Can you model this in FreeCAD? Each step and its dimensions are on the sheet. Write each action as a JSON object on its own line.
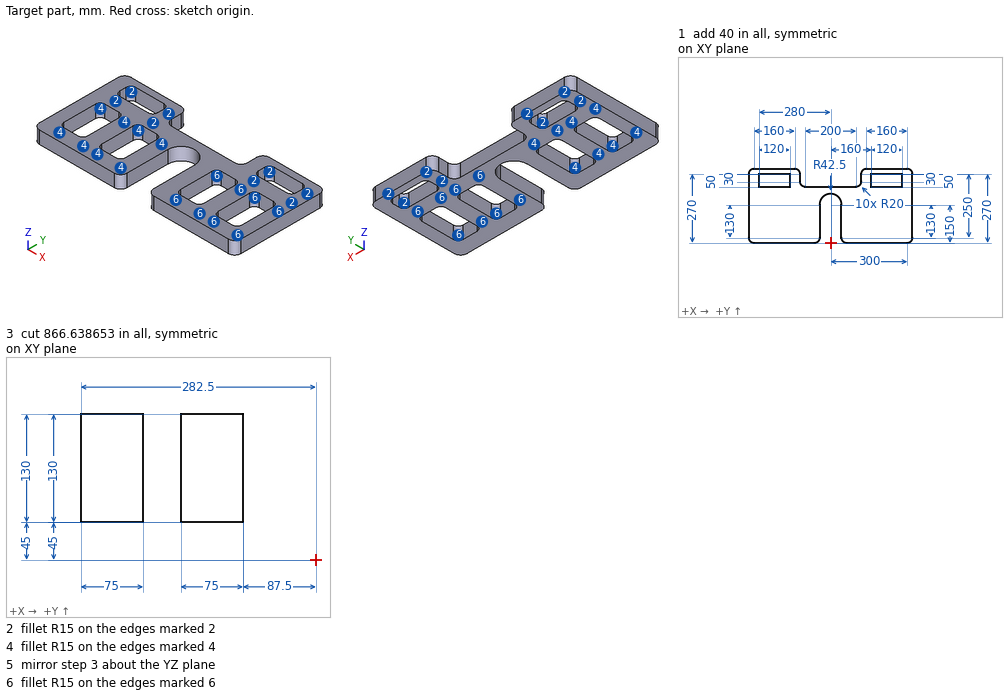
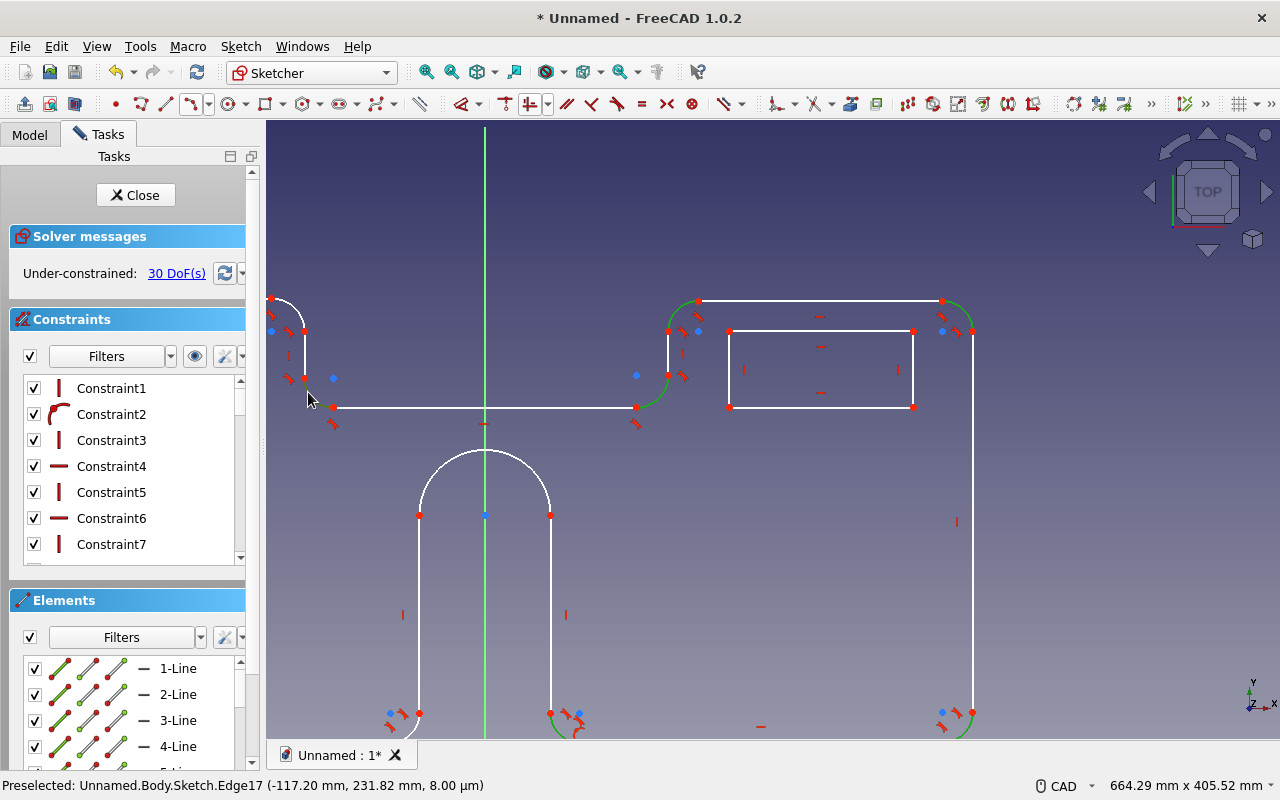
{"action": "left_click", "coordinate": [301, 316]}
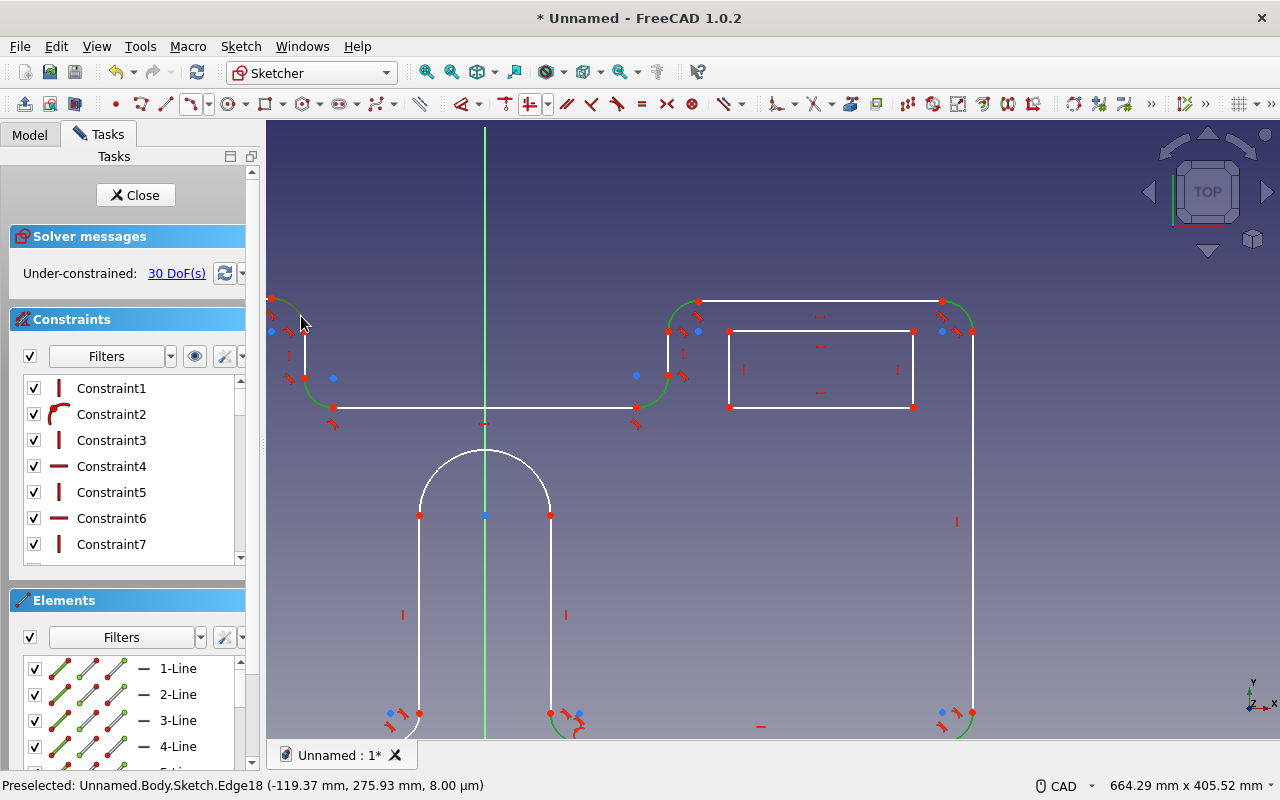
{"action": "scroll", "coordinate": [971, 318], "scroll_direction": "down", "scroll_amount": 3}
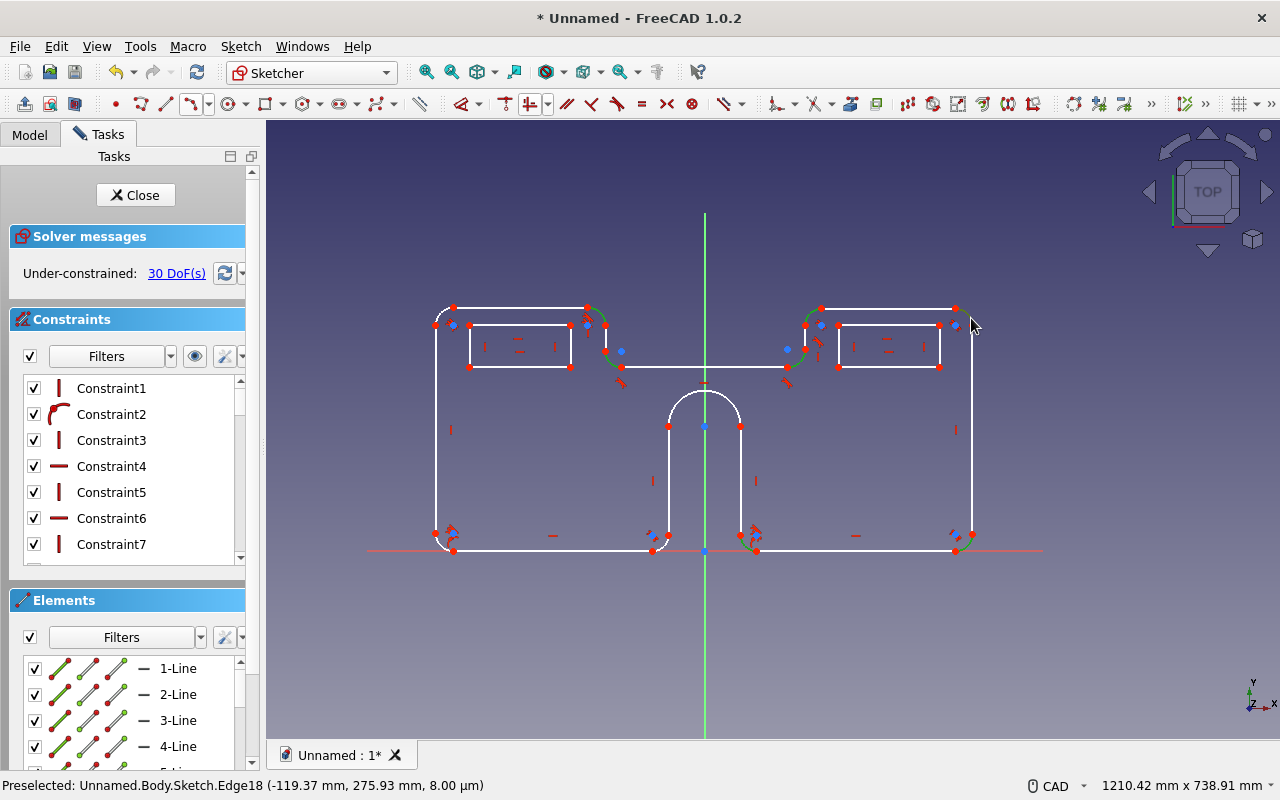
{"action": "scroll", "coordinate": [446, 309], "scroll_direction": "up", "scroll_amount": 3}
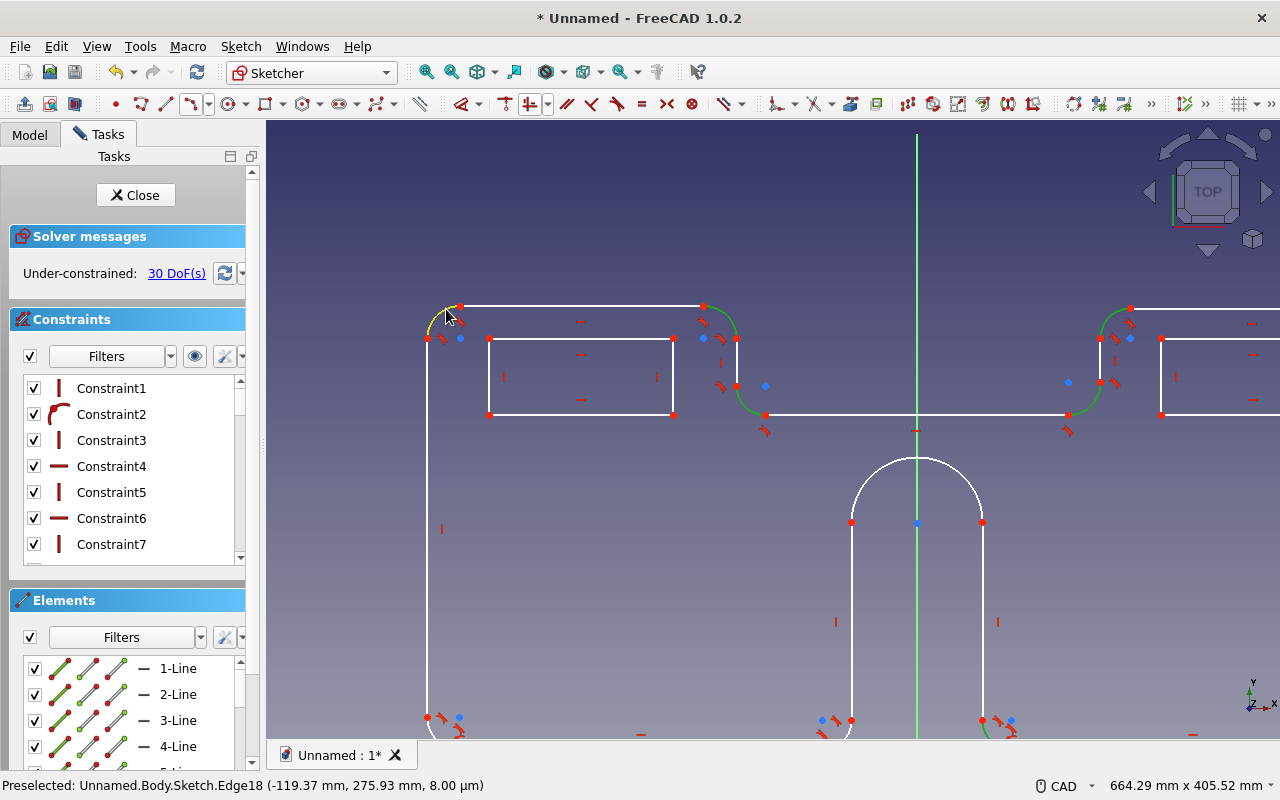
{"action": "left_click", "coordinate": [445, 310]}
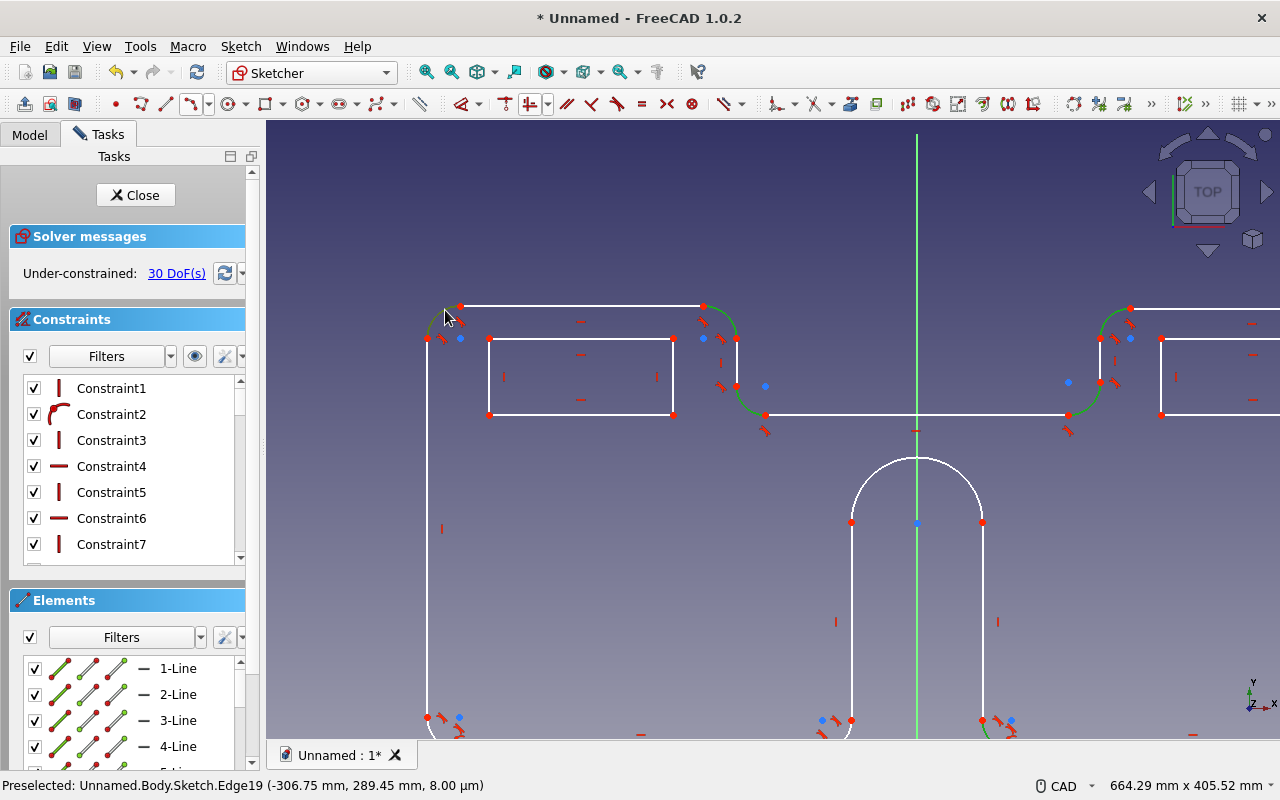
{"action": "scroll", "coordinate": [446, 309], "scroll_direction": "down", "scroll_amount": 3}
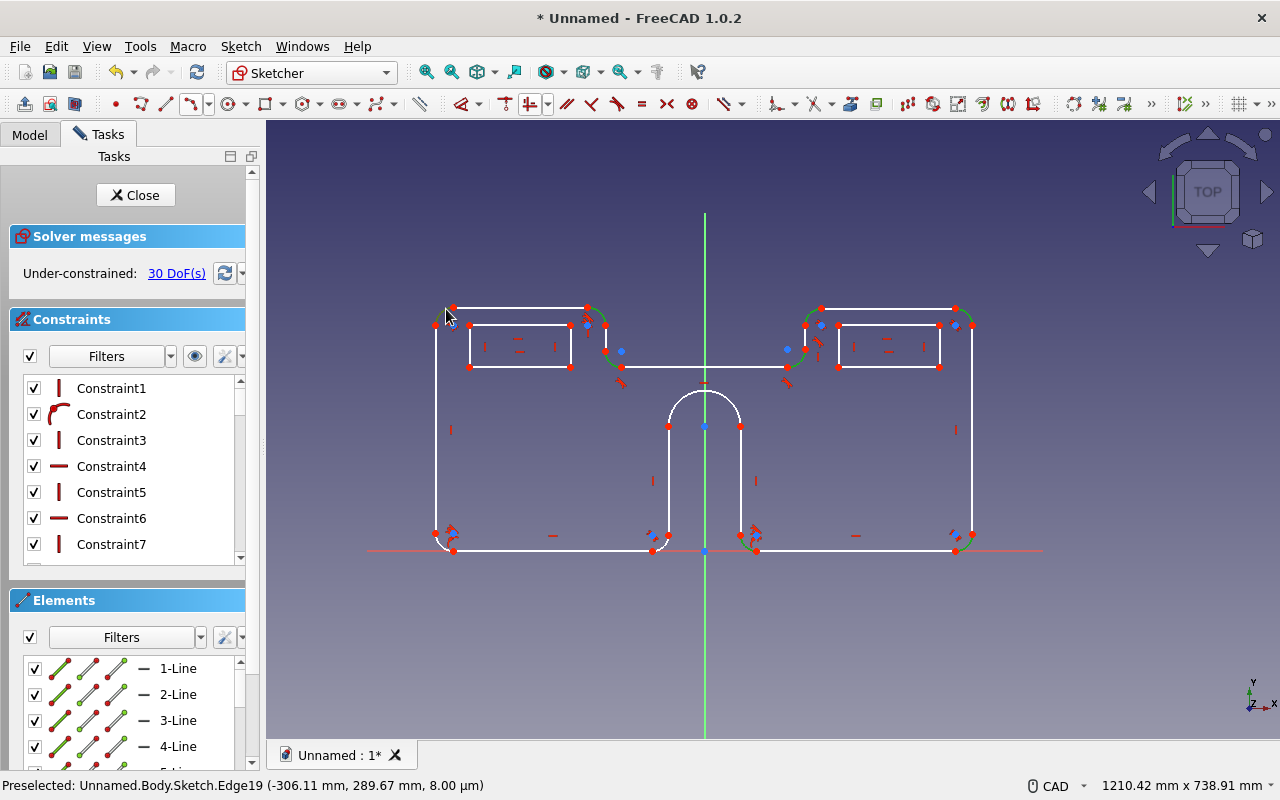
{"action": "scroll", "coordinate": [438, 541], "scroll_direction": "up", "scroll_amount": 3}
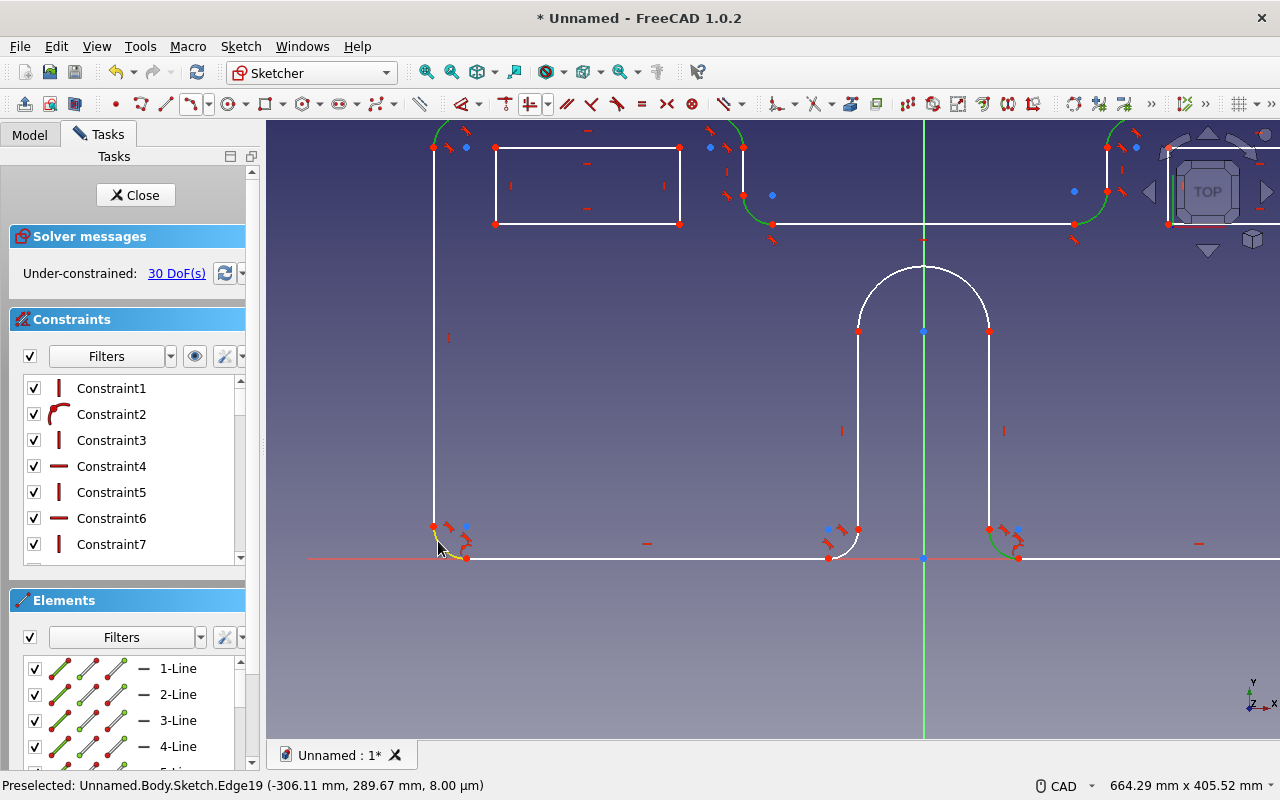
{"action": "left_click", "coordinate": [437, 541]}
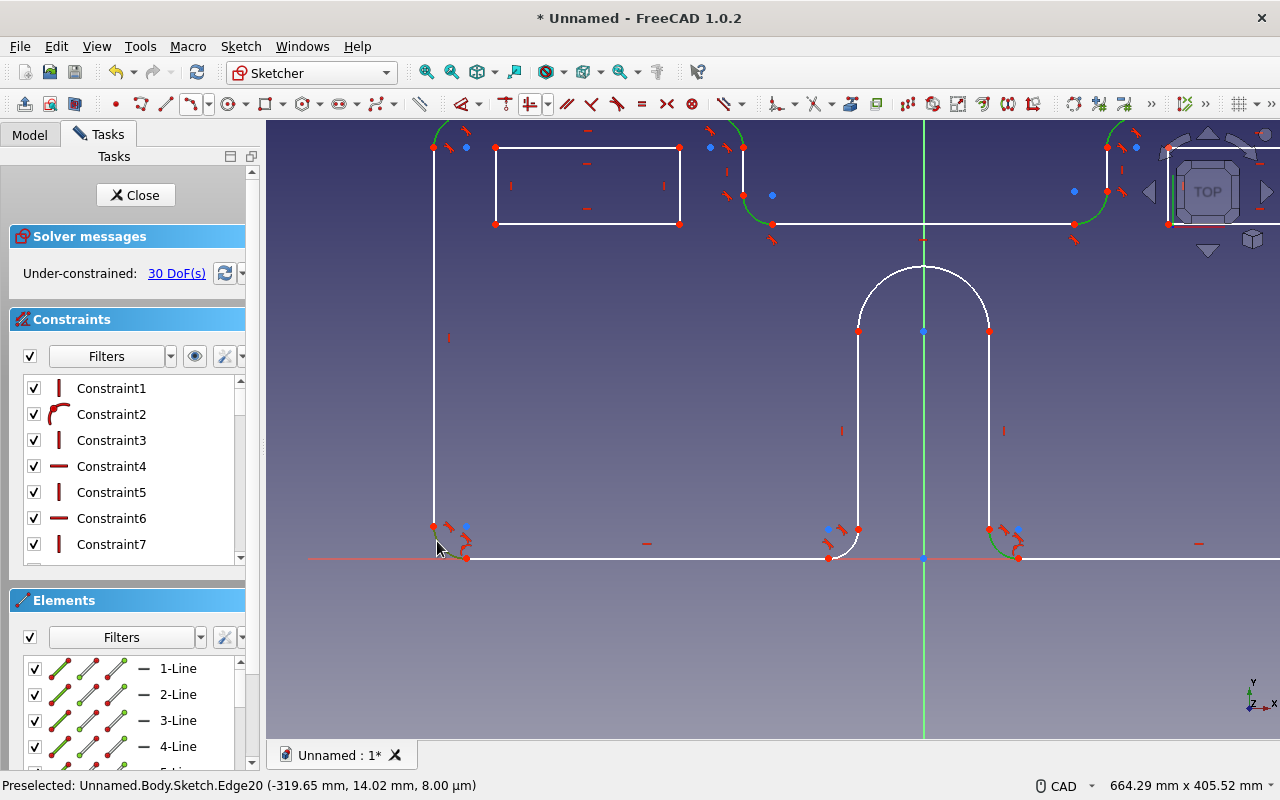
{"action": "left_click", "coordinate": [842, 556]}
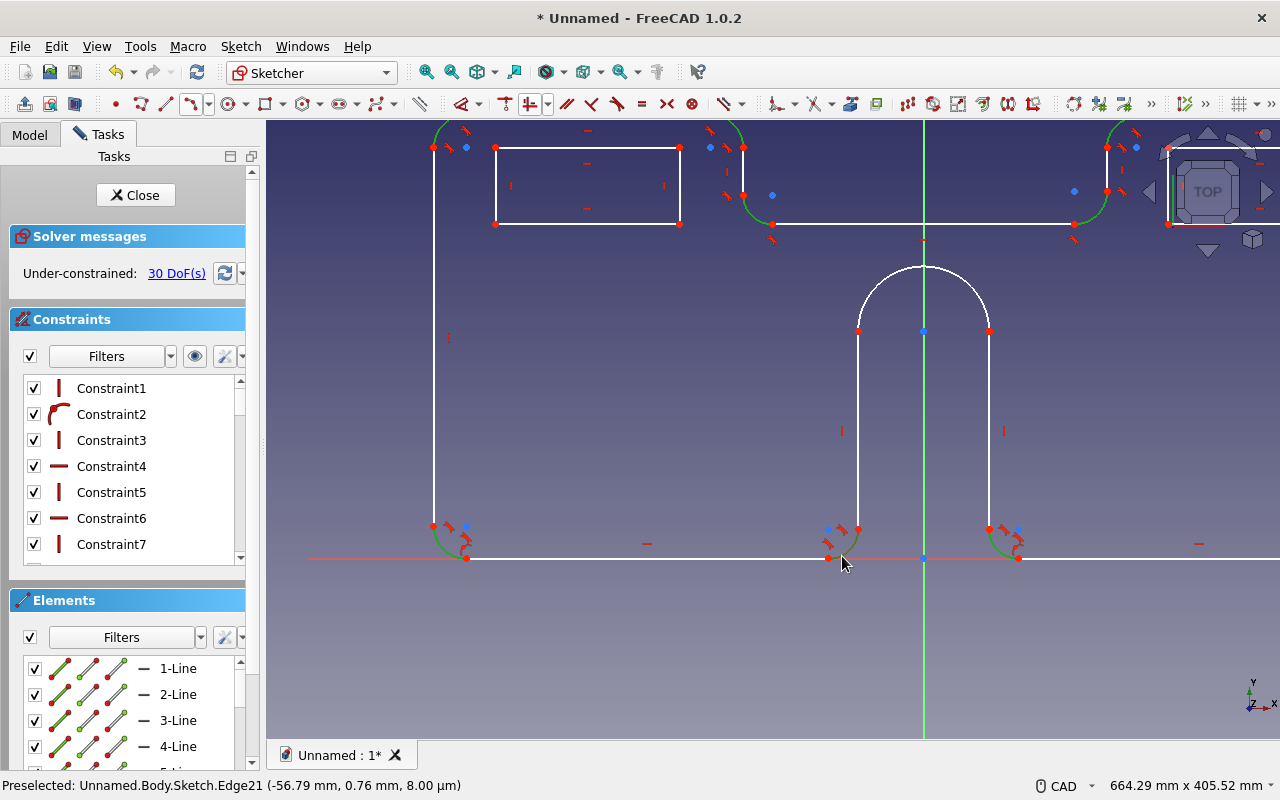
{"action": "key", "text": "e"}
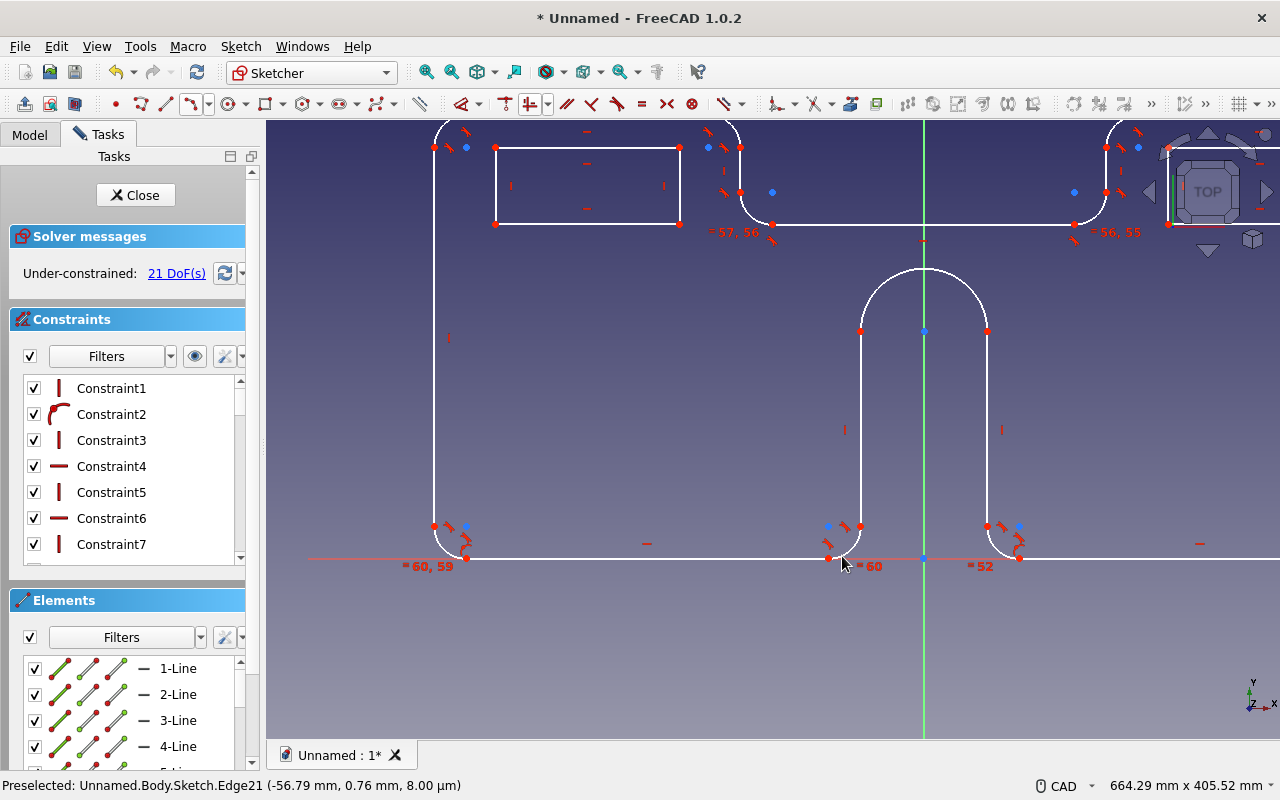
{"action": "left_click", "coordinate": [924, 332]}